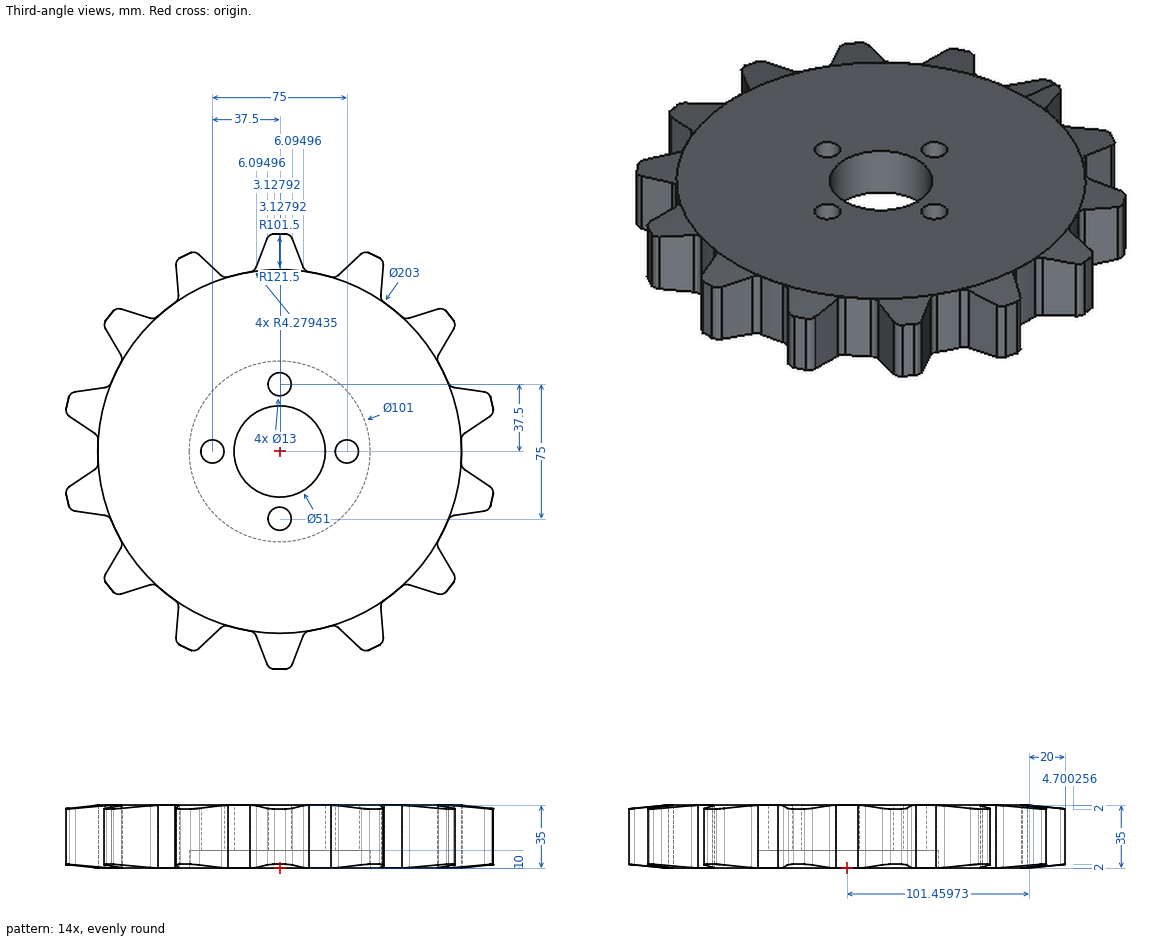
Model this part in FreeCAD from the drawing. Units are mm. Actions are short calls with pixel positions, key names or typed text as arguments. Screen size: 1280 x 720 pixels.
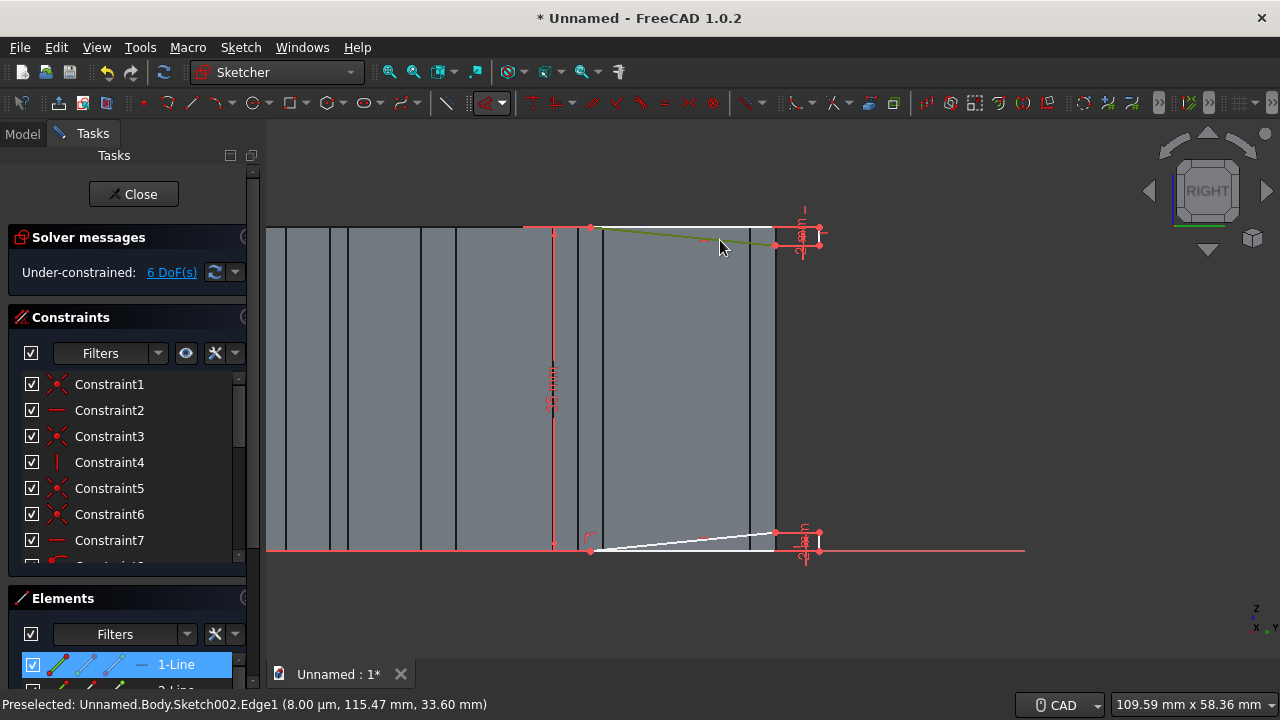
click(504, 104)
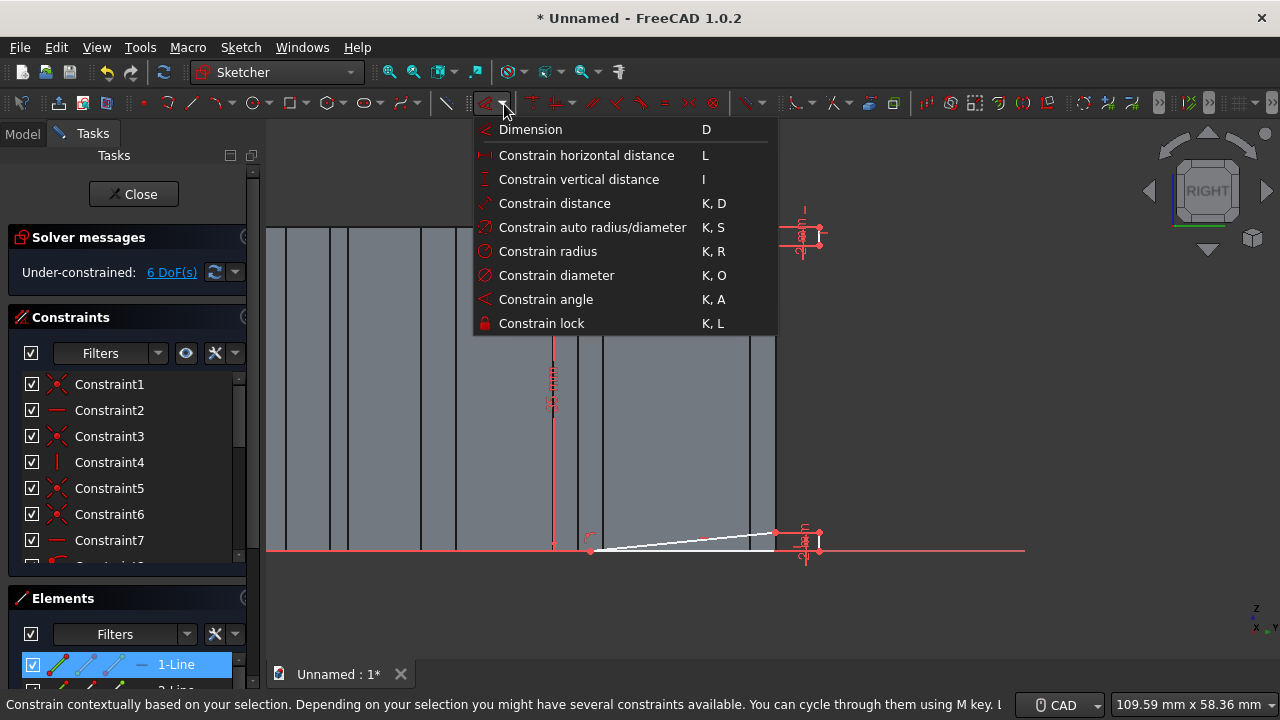
click(626, 155)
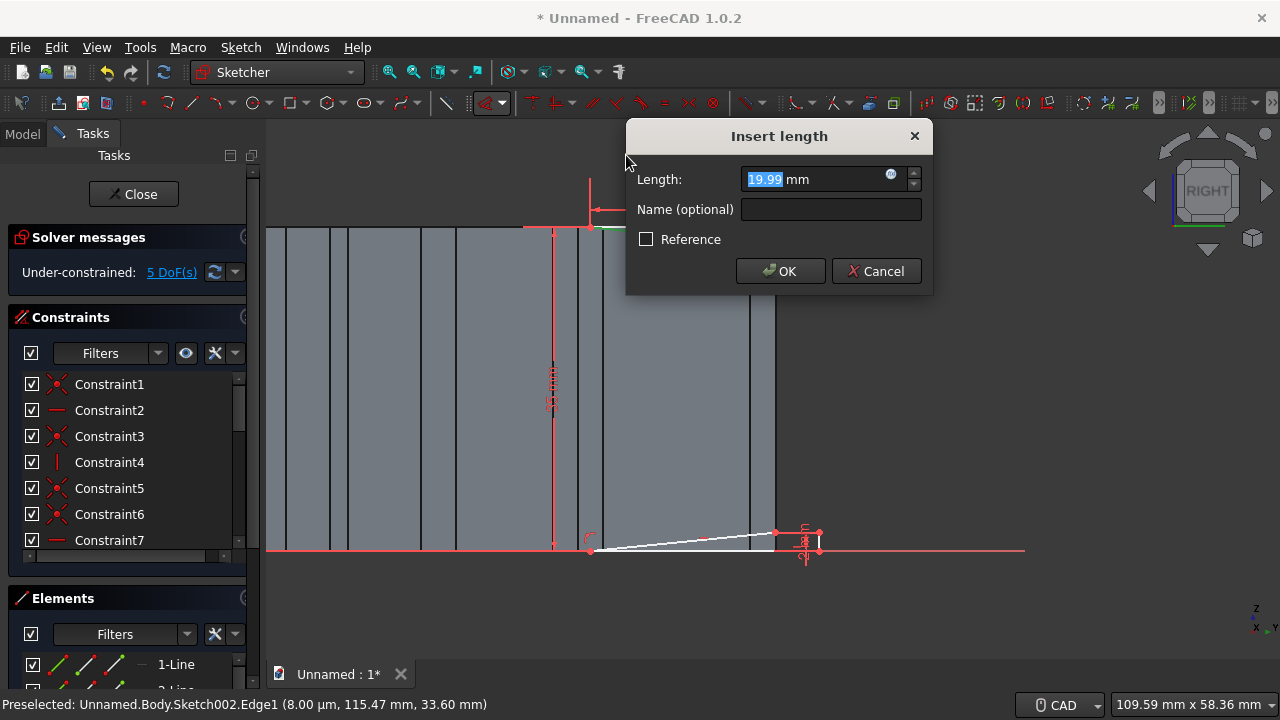
text(20)
key(Return)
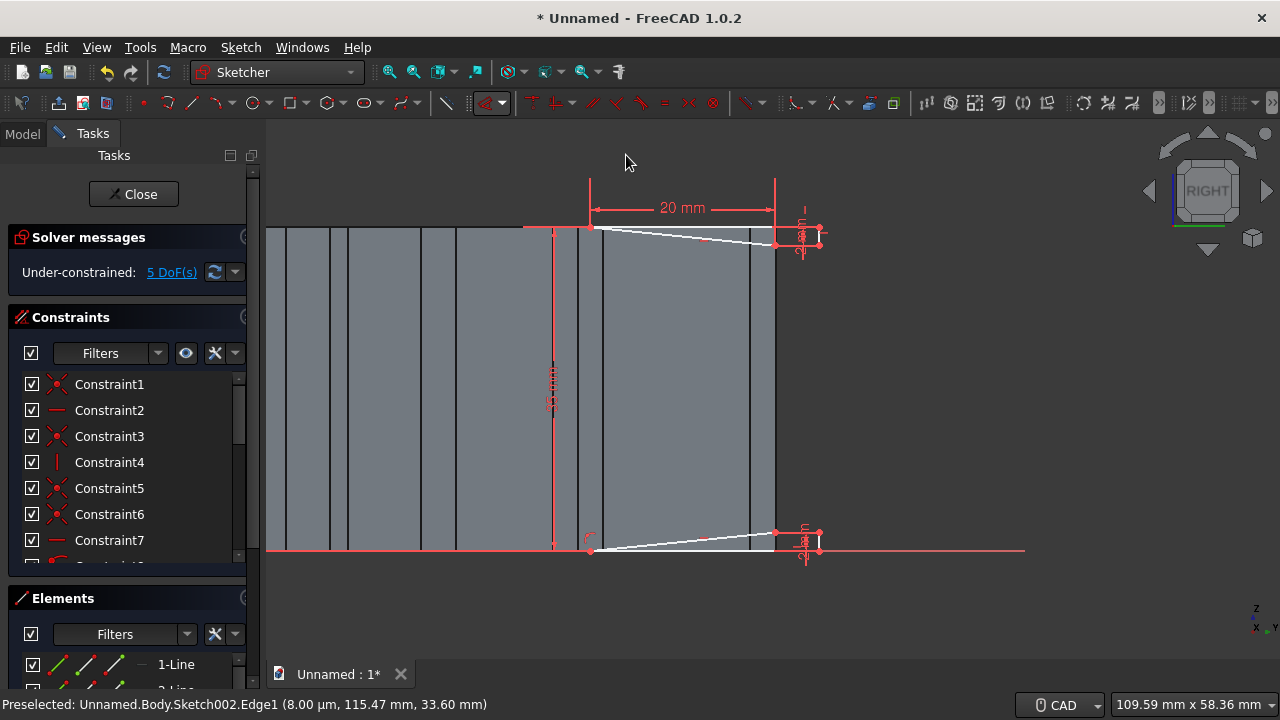
click(720, 538)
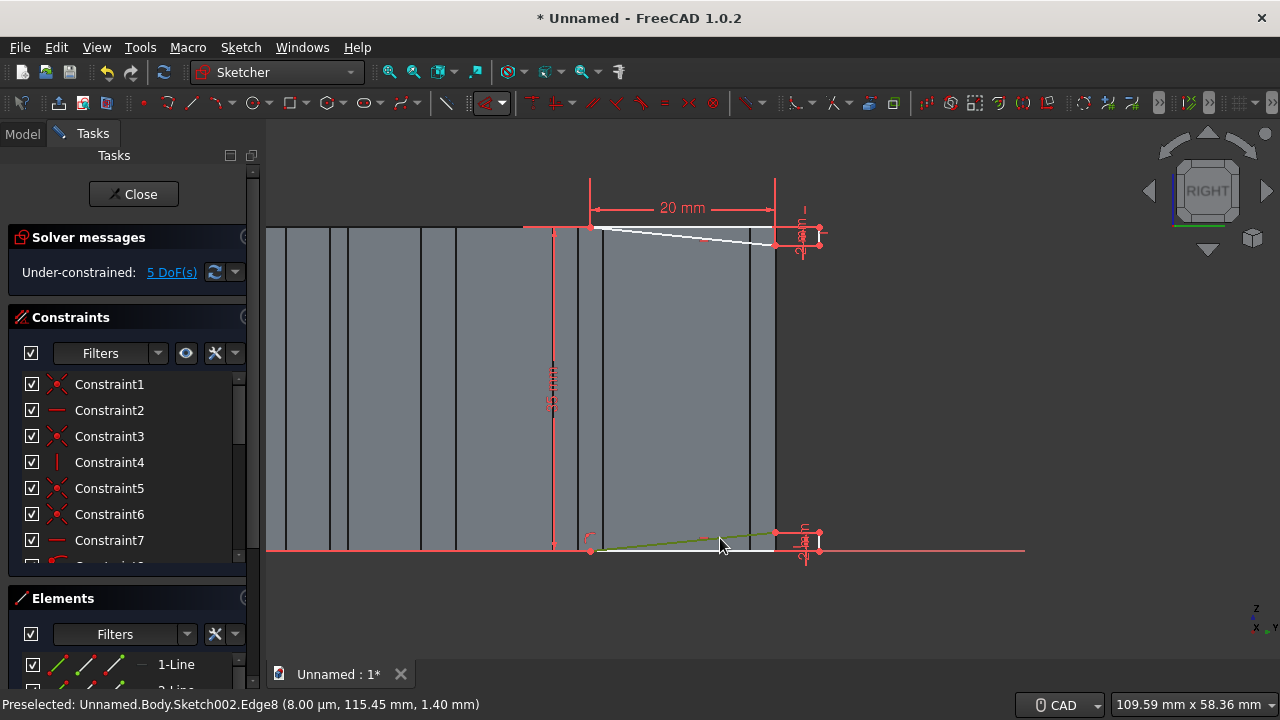
click(504, 104)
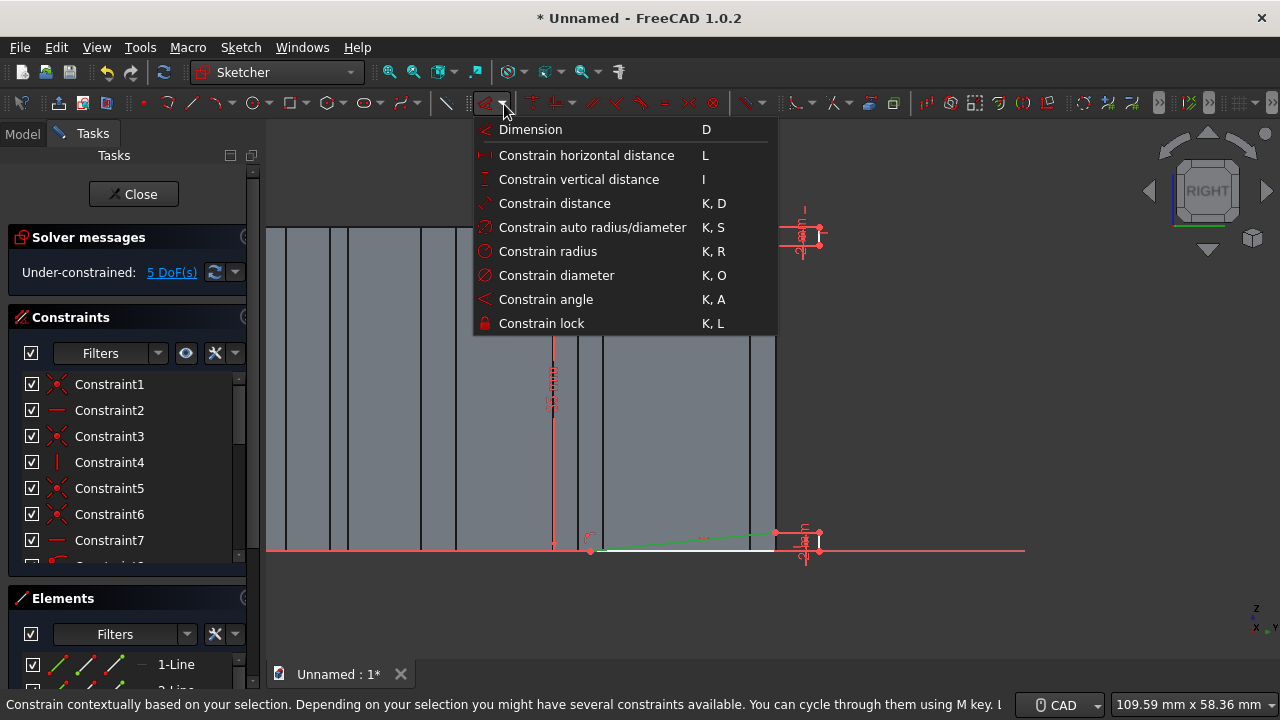
click(626, 155)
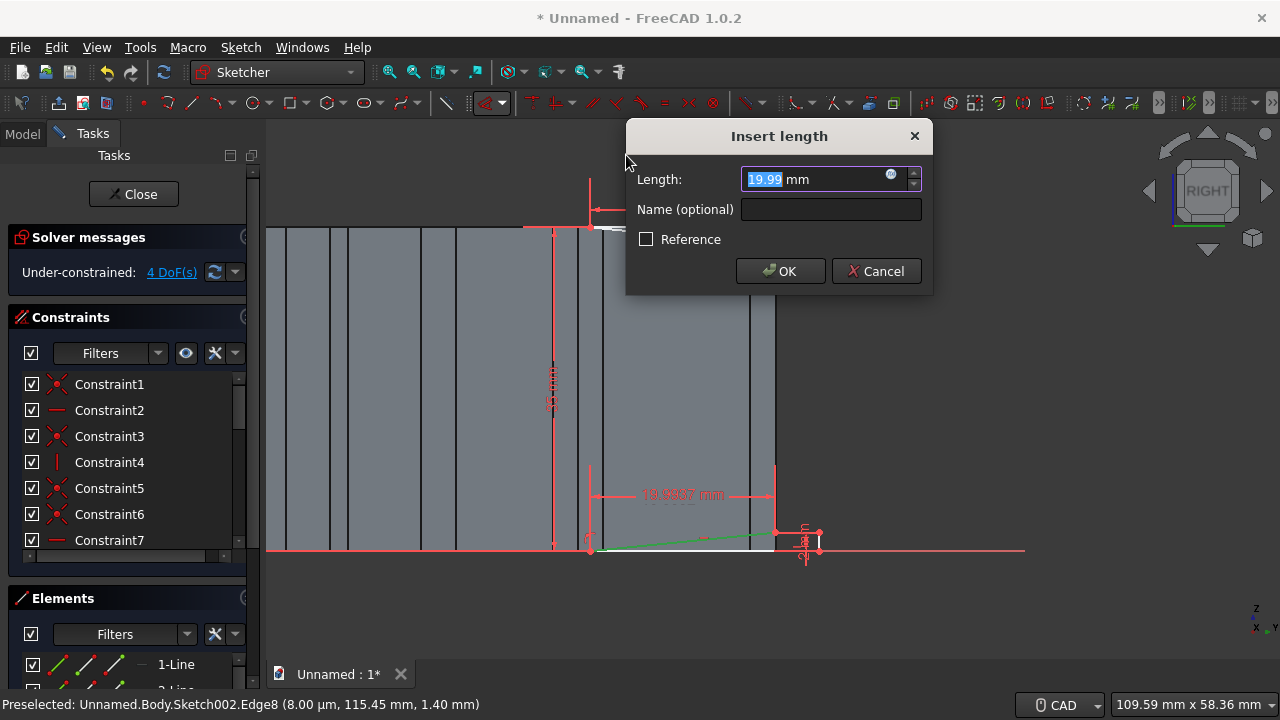
text(20)
key(Return)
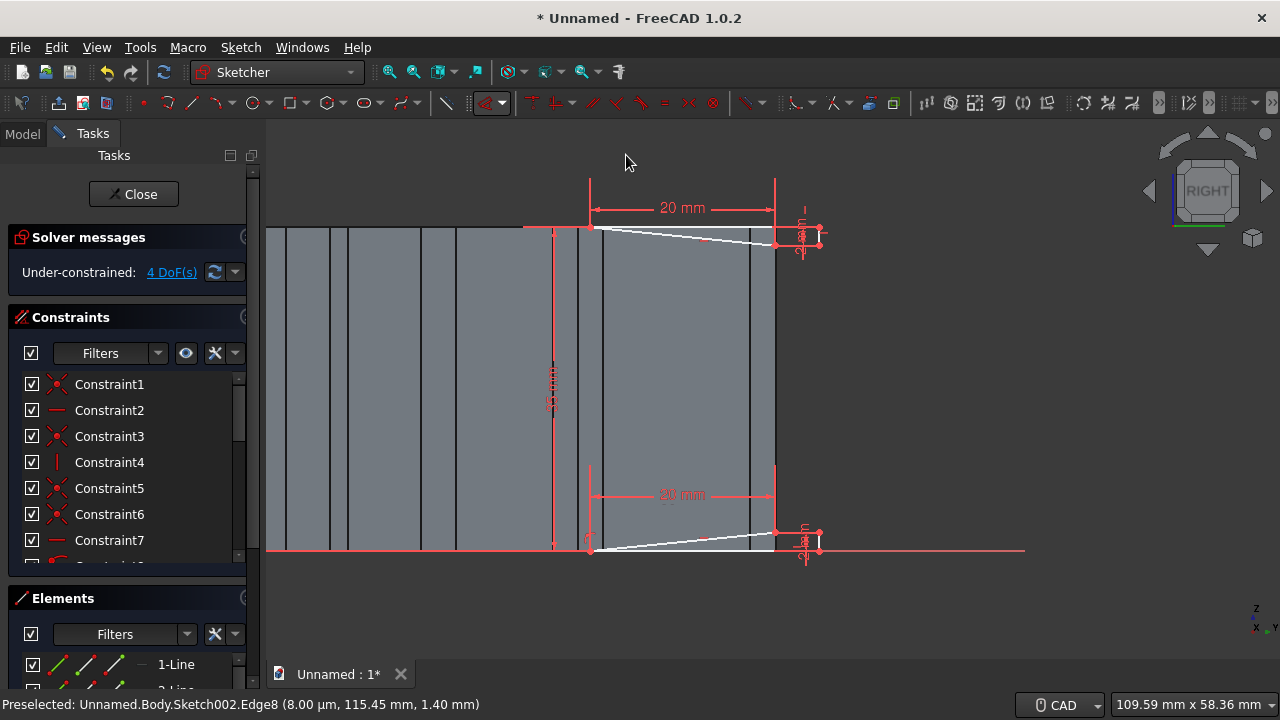
click(789, 246)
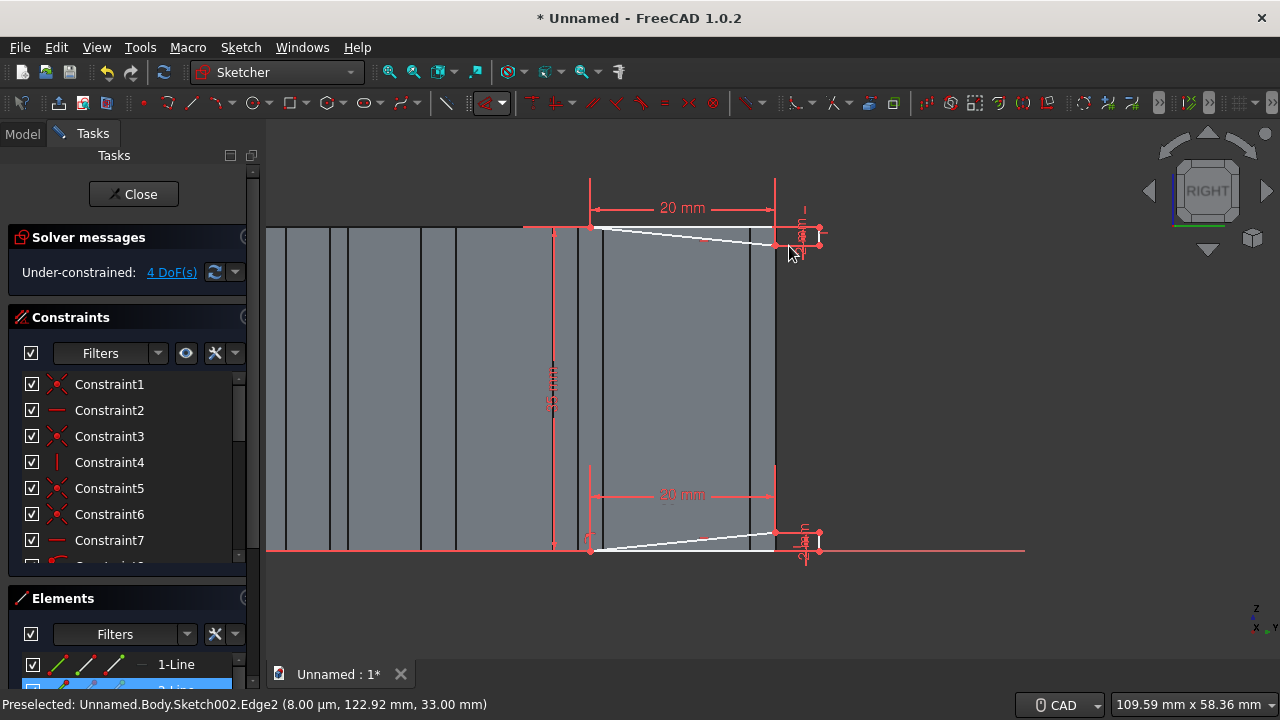
click(504, 104)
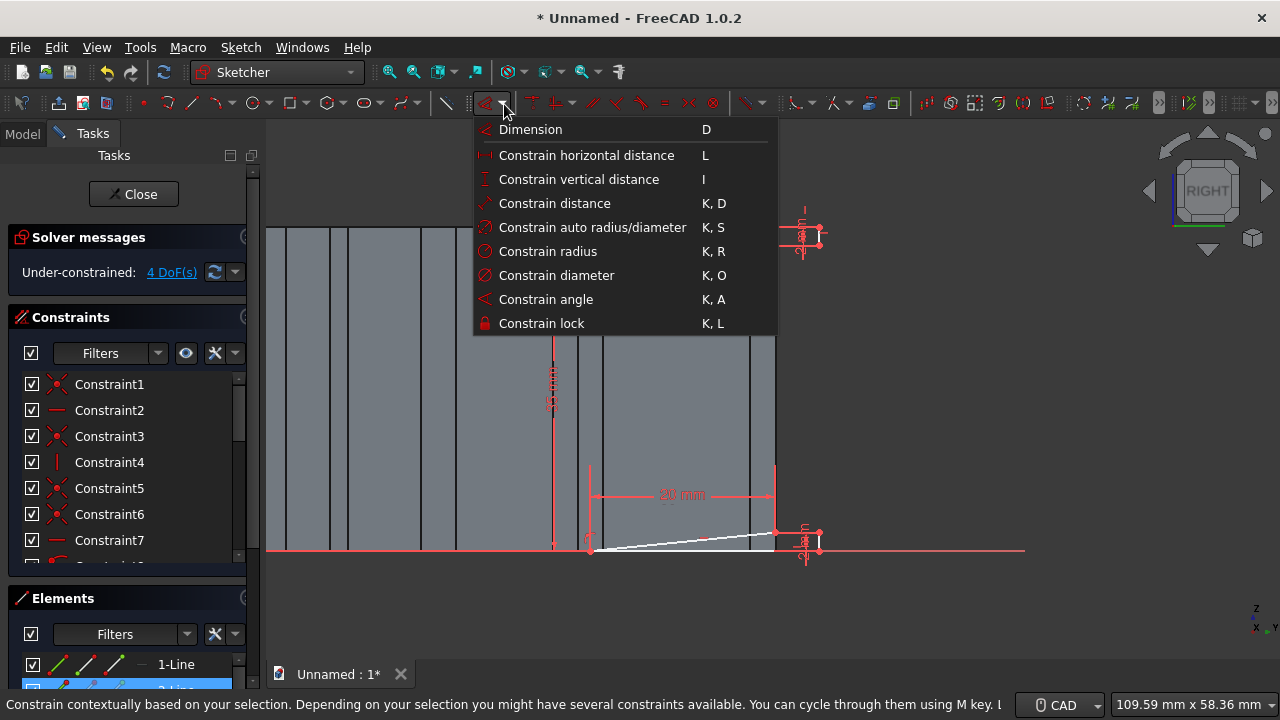
click(626, 155)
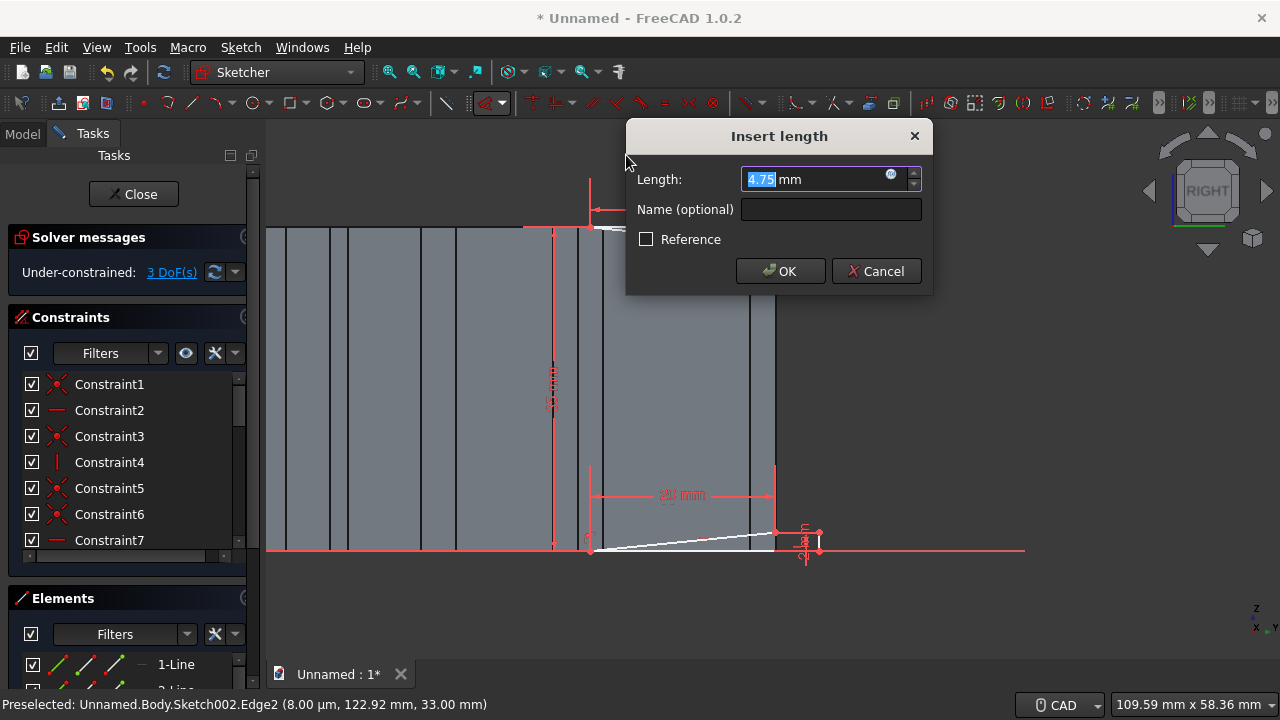
text(4.700256)
key(Return)